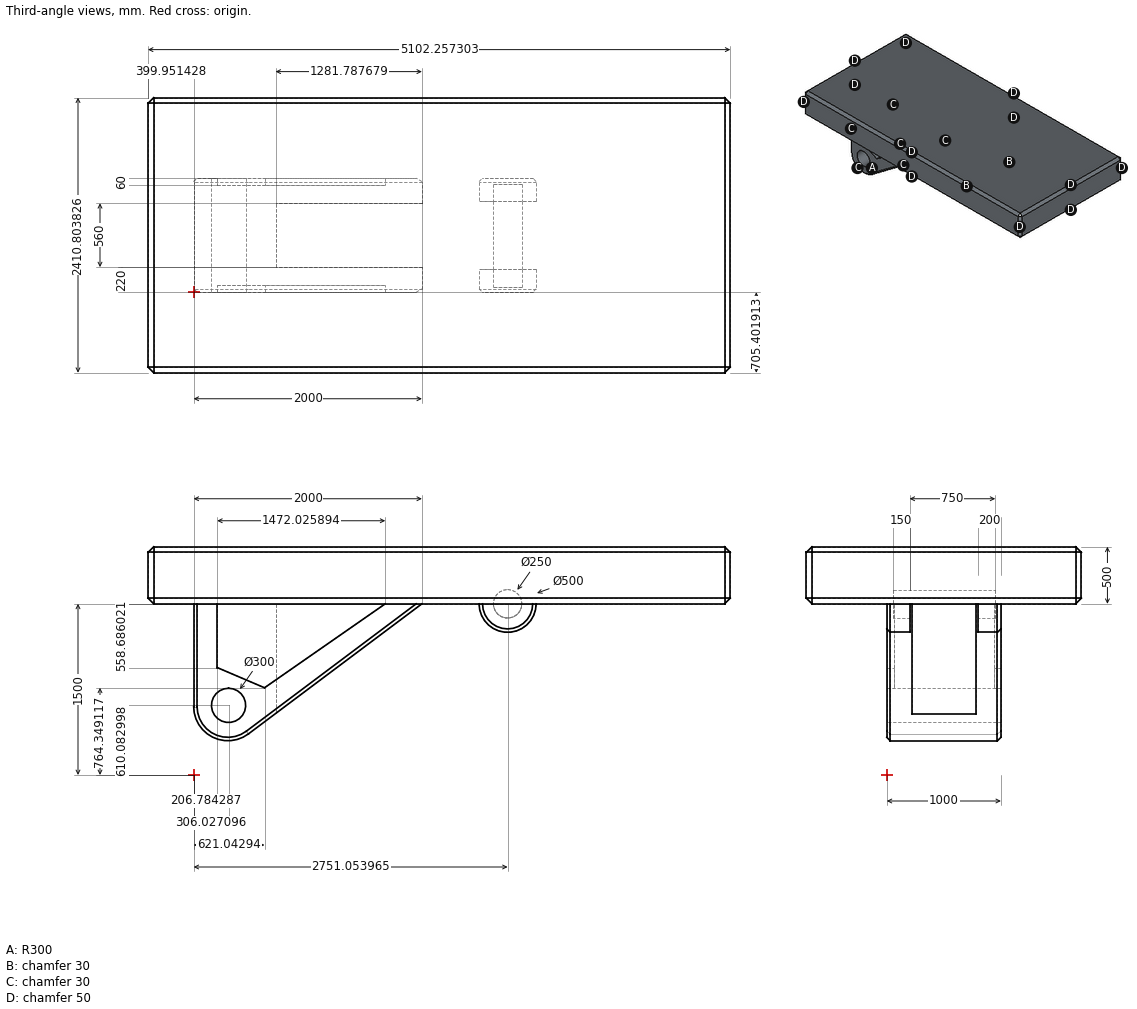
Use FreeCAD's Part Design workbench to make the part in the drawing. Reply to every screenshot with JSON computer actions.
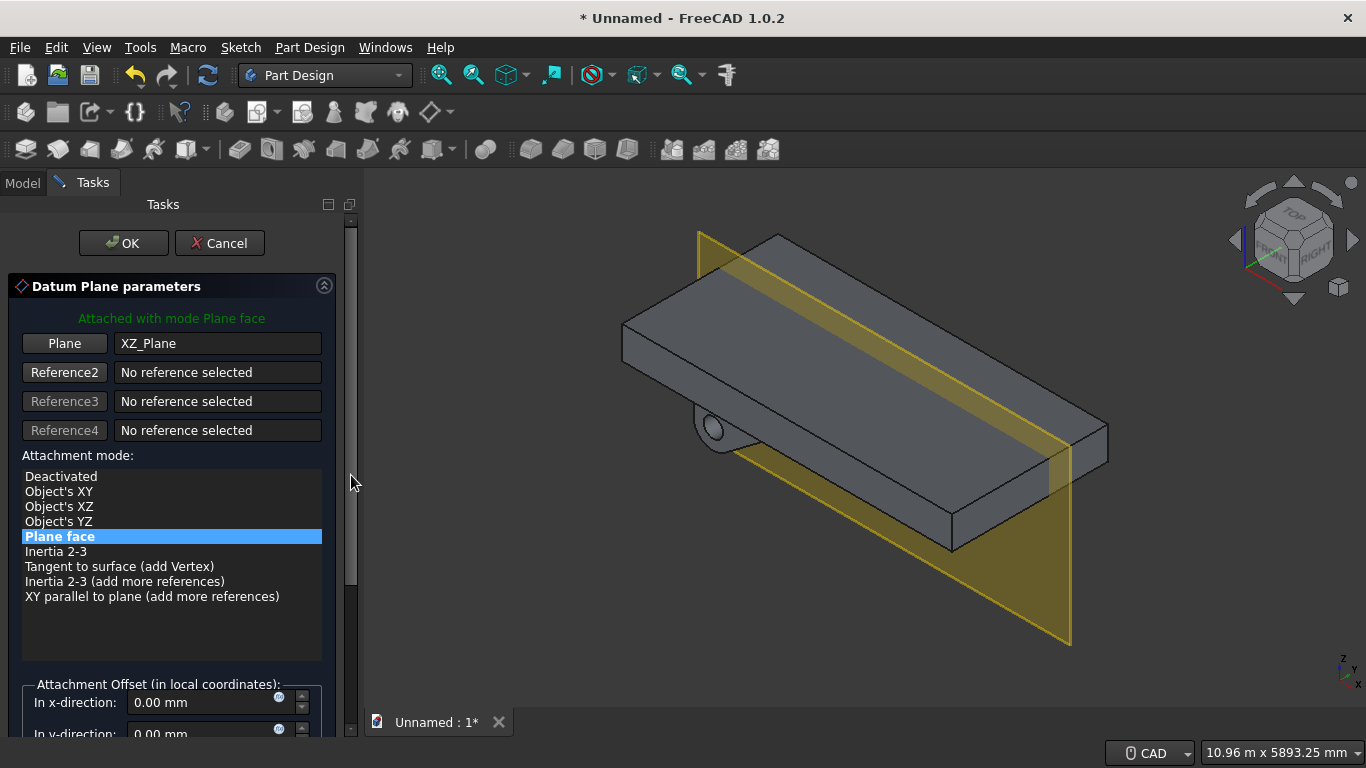
{"action": "left_click", "coordinate": [124, 243]}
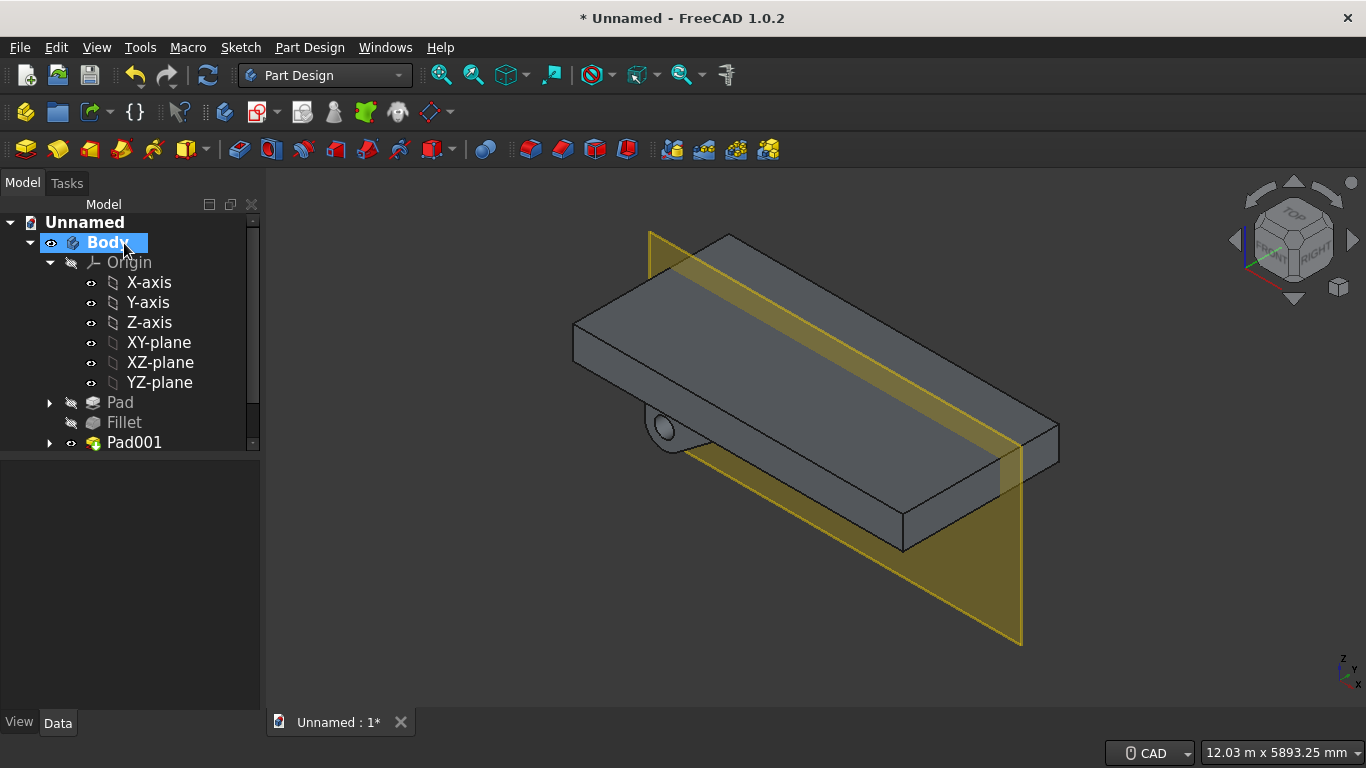
{"action": "scroll", "coordinate": [100, 338], "scroll_direction": "down", "scroll_amount": 3}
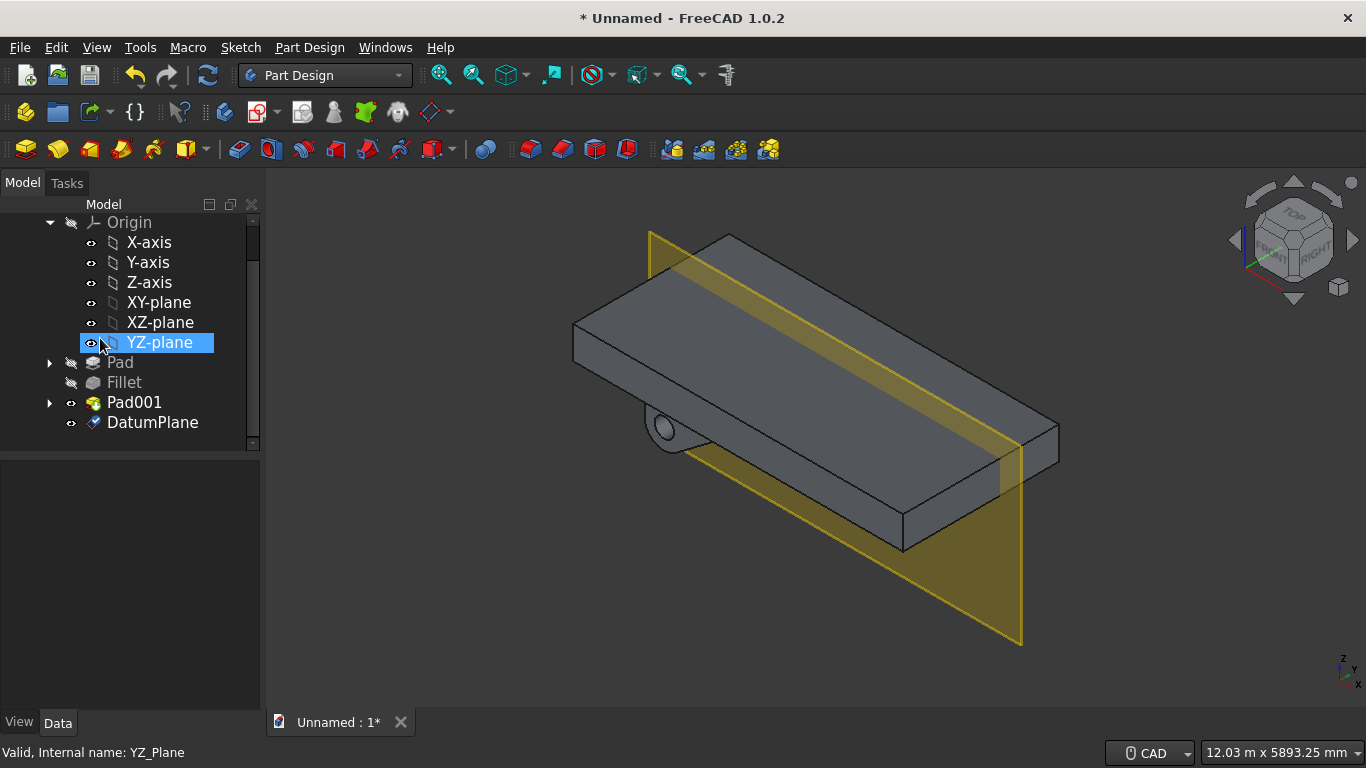
{"action": "left_click", "coordinate": [116, 423]}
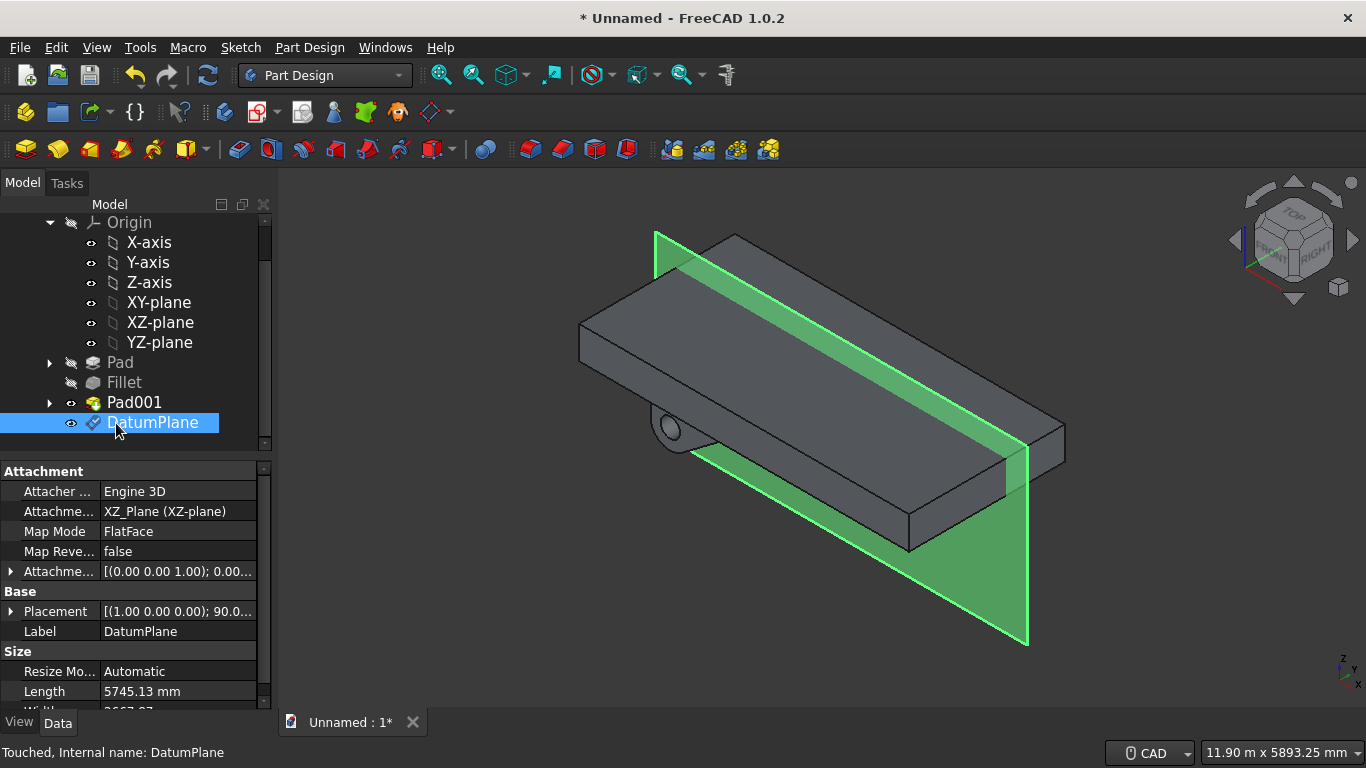
{"action": "left_click", "coordinate": [258, 112]}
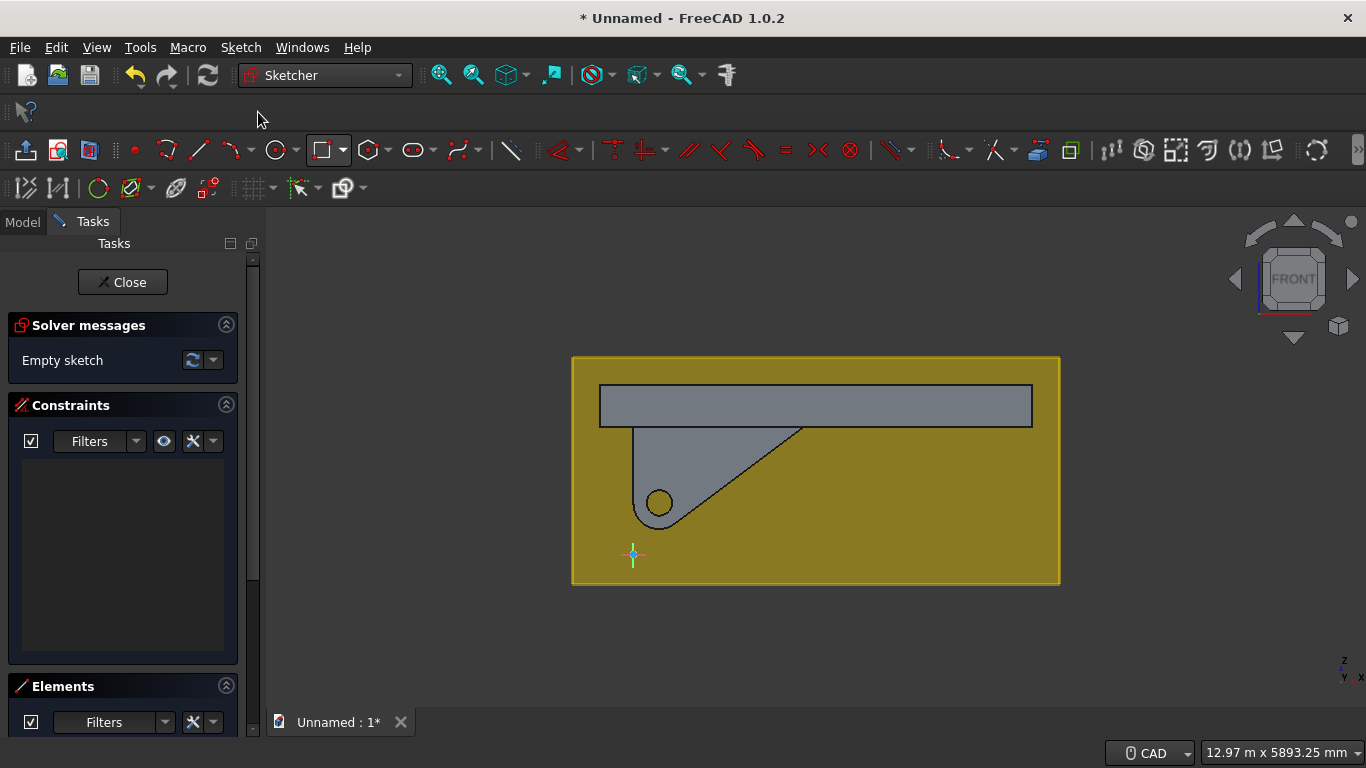
{"action": "left_click", "coordinate": [90, 150]}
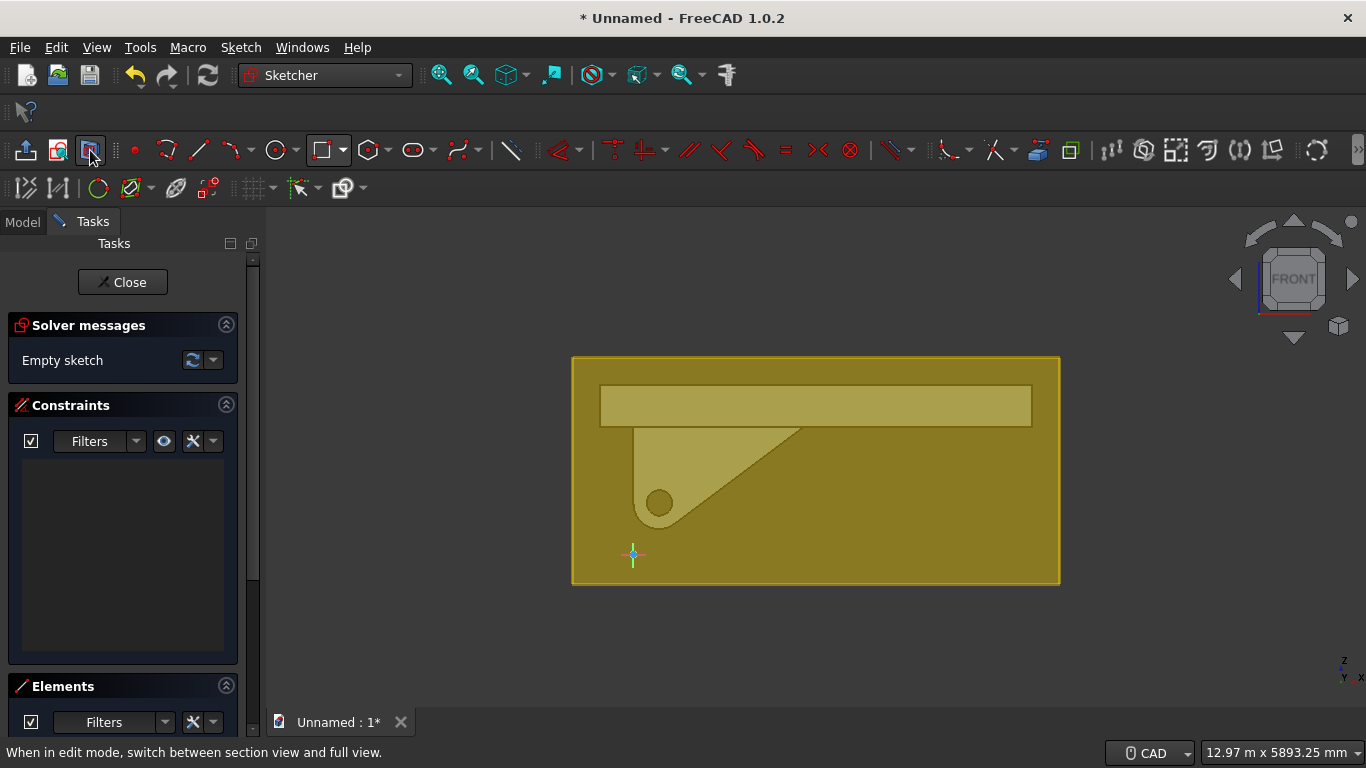
{"action": "scroll", "coordinate": [886, 423], "scroll_direction": "up", "scroll_amount": 10}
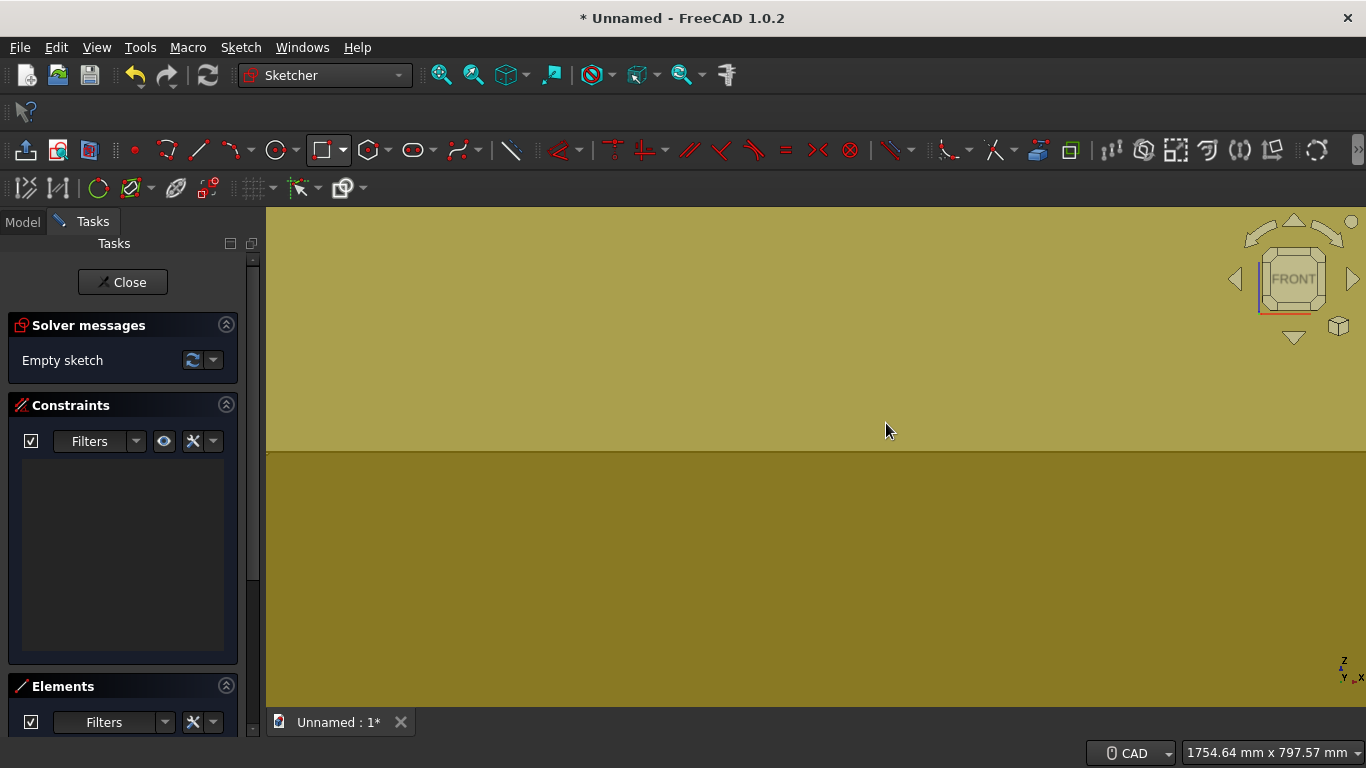
{"action": "left_click", "coordinate": [276, 150]}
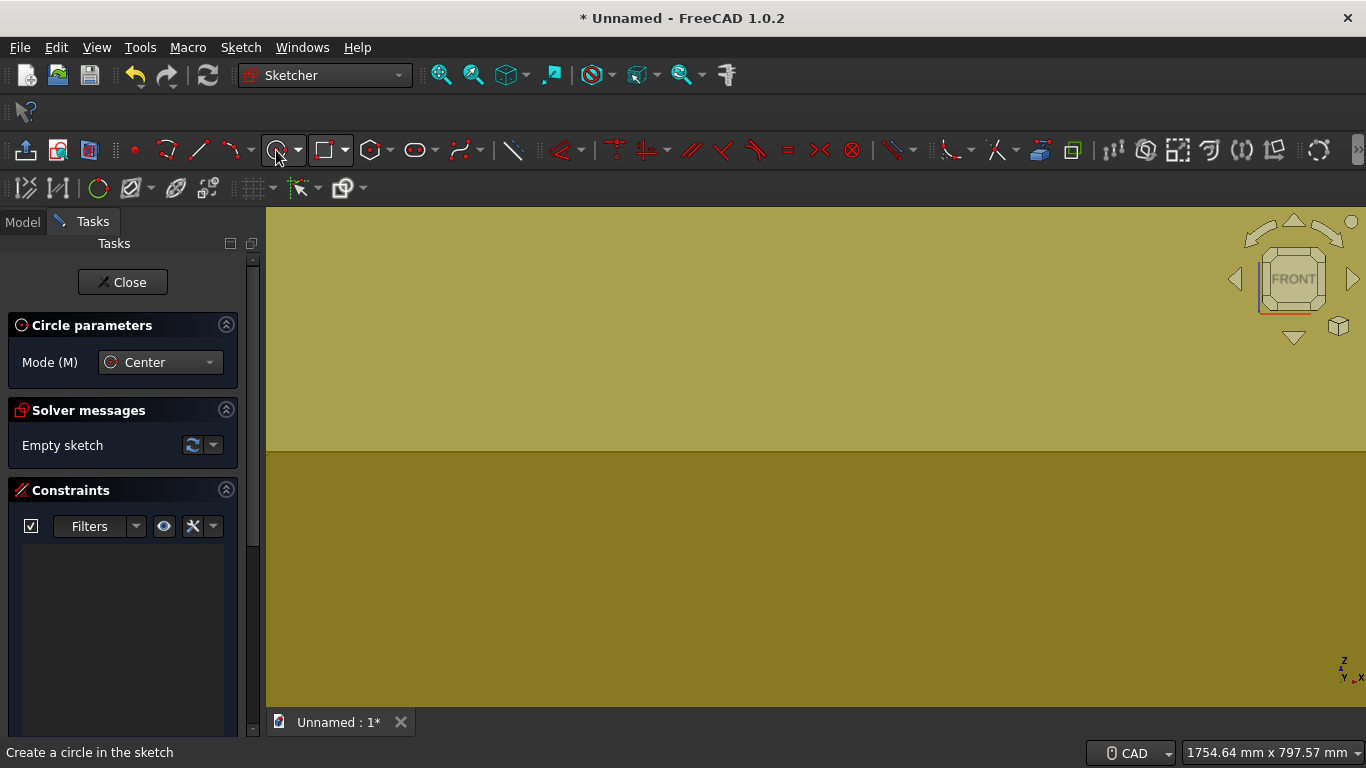
{"action": "left_click", "coordinate": [741, 452]}
{"action": "mouse_move", "coordinate": [852, 342]}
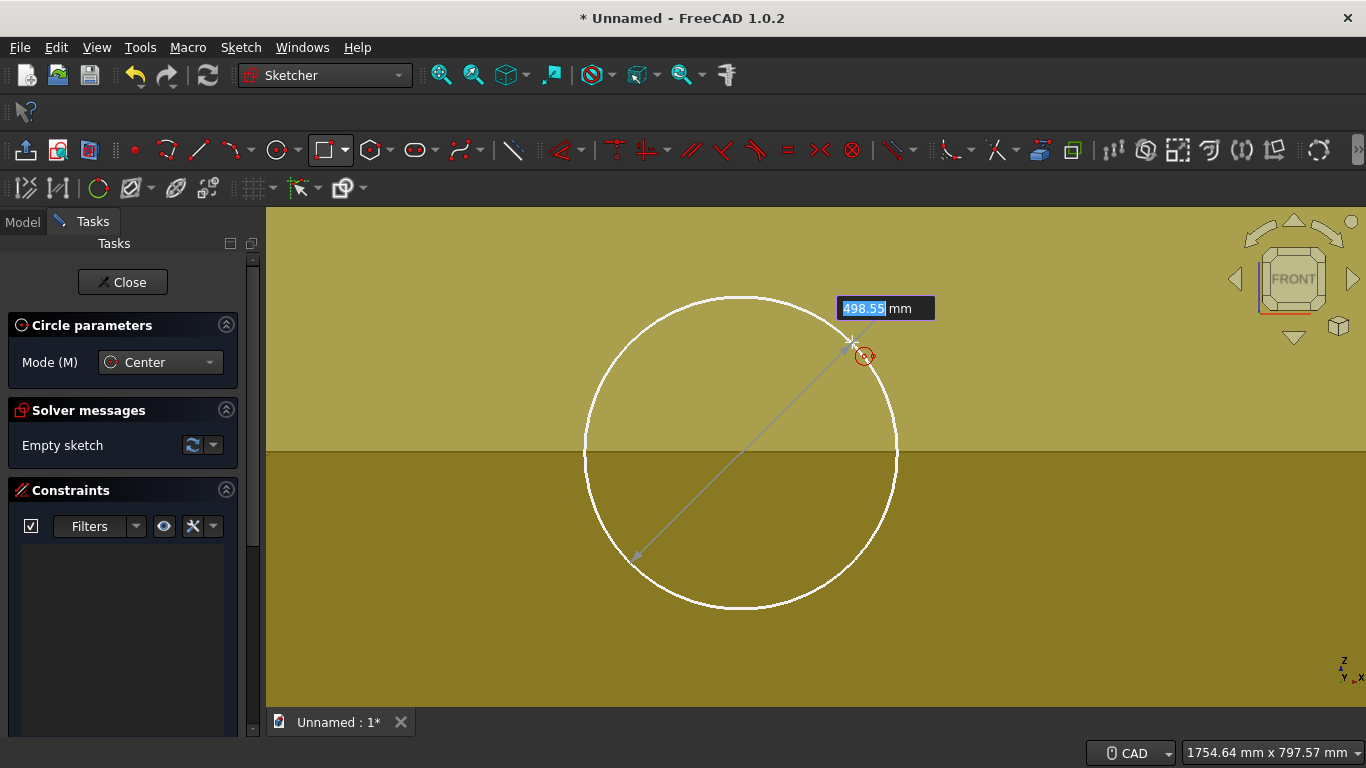
{"action": "type", "text": "500"}
{"action": "key", "text": "Return"}
{"action": "key", "text": "Escape"}